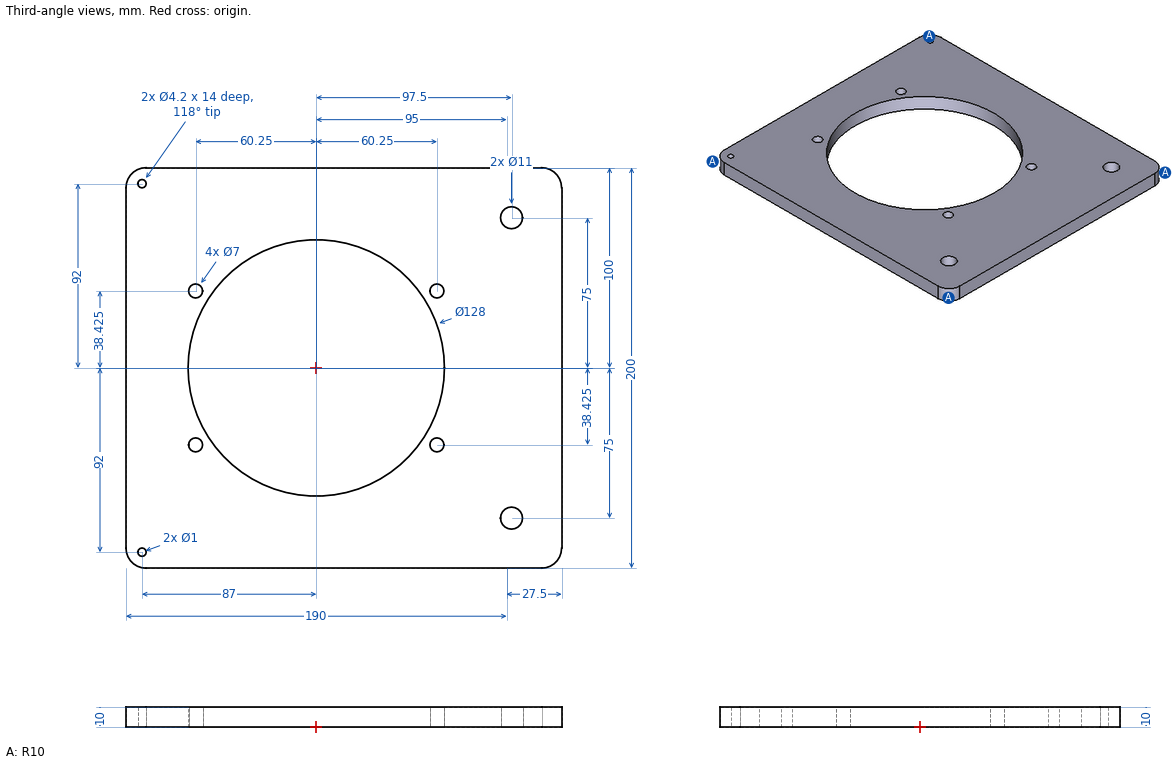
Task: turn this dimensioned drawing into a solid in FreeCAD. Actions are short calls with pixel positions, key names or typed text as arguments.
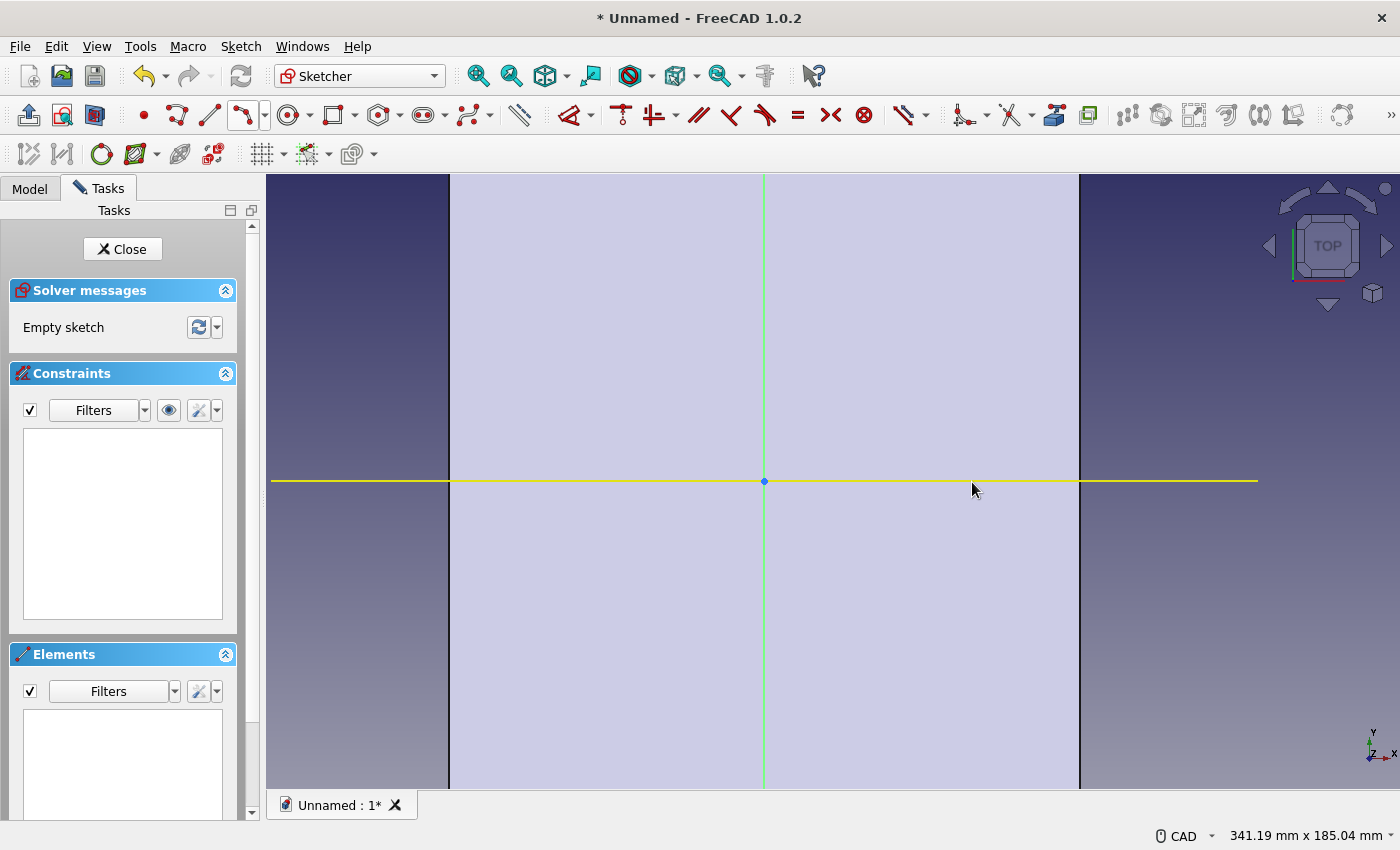
key(g)
key(c)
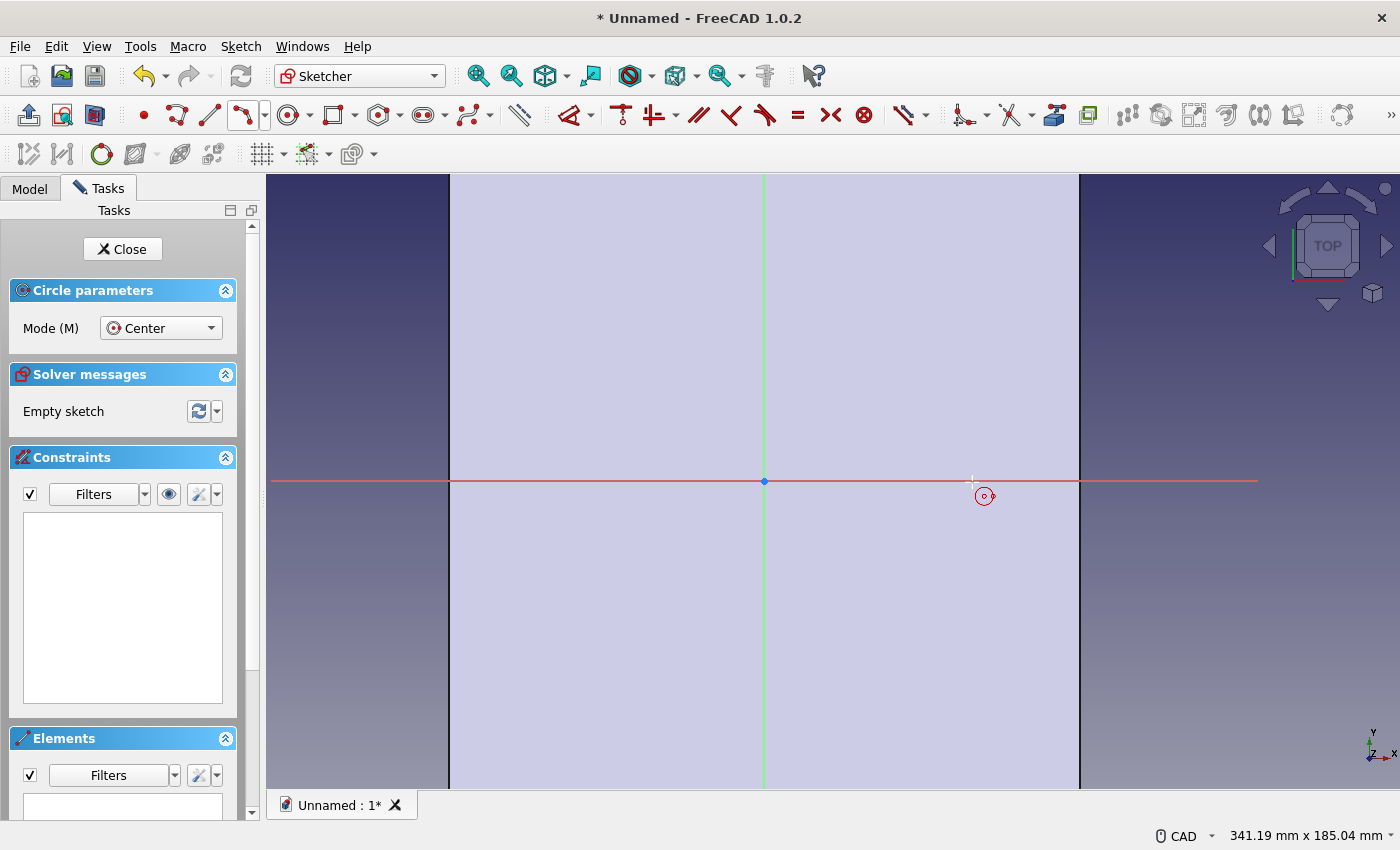
click(764, 481)
move(915, 331)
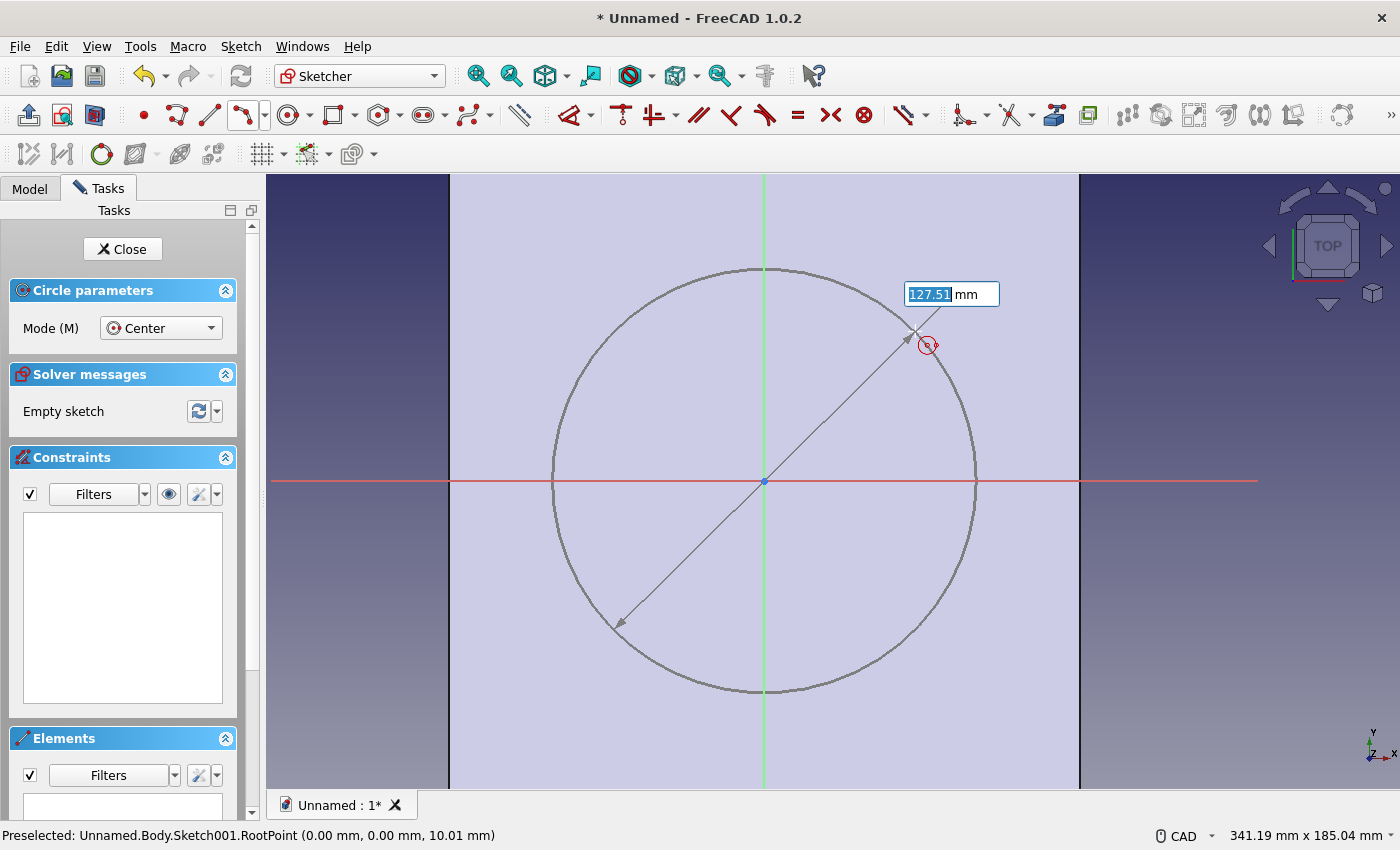
text(128)
key(Return)
key(Escape)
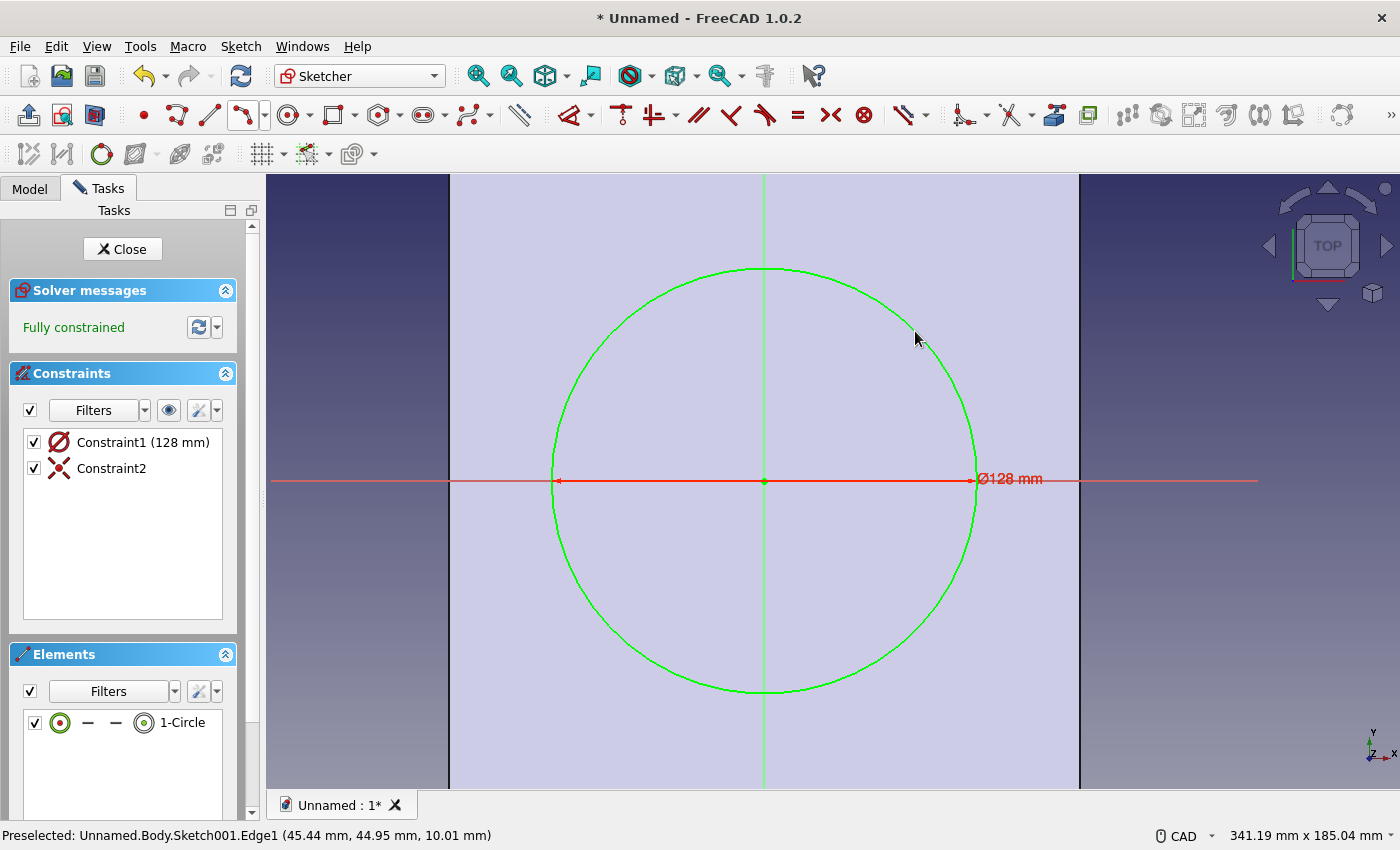
click(123, 249)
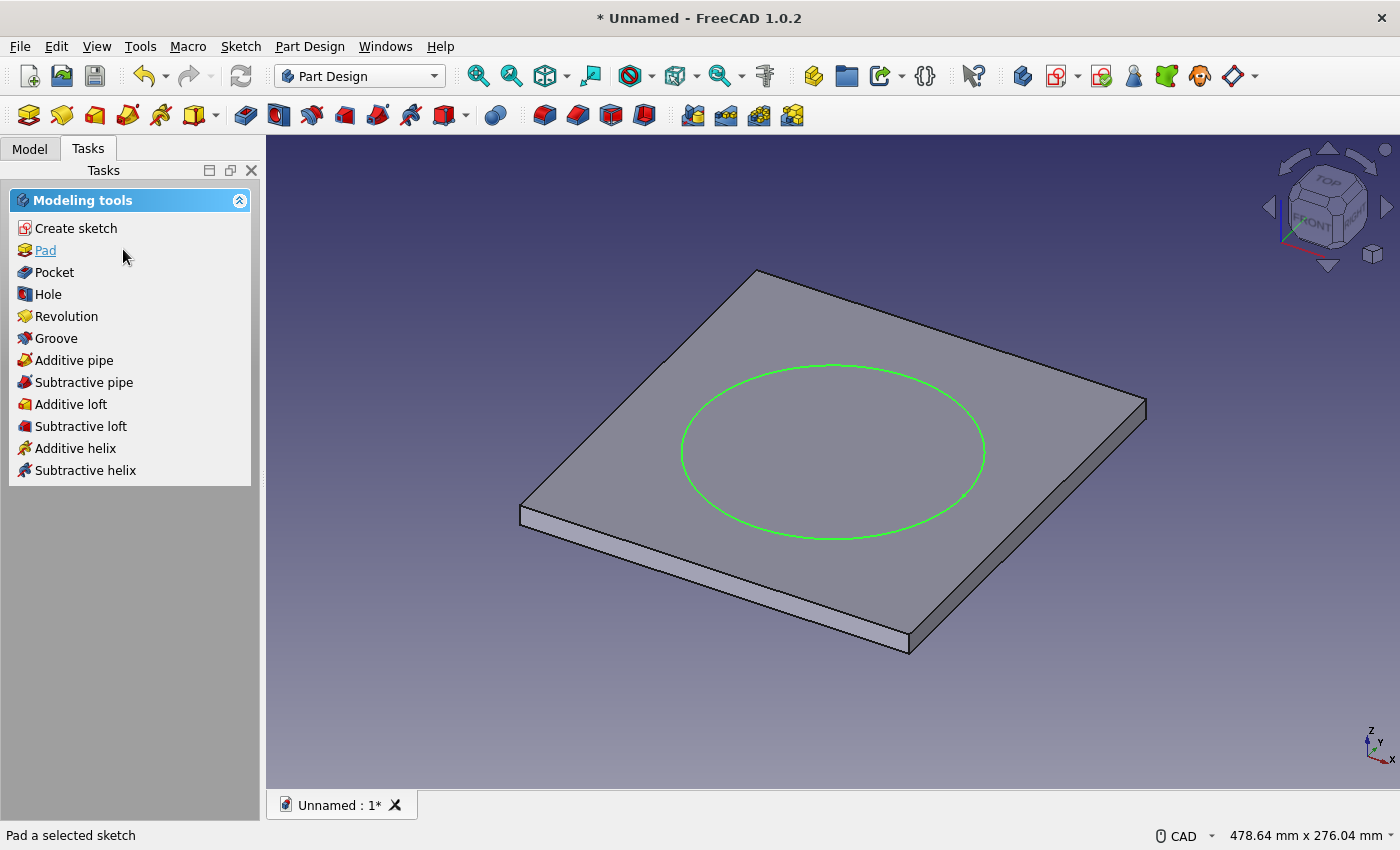
click(246, 116)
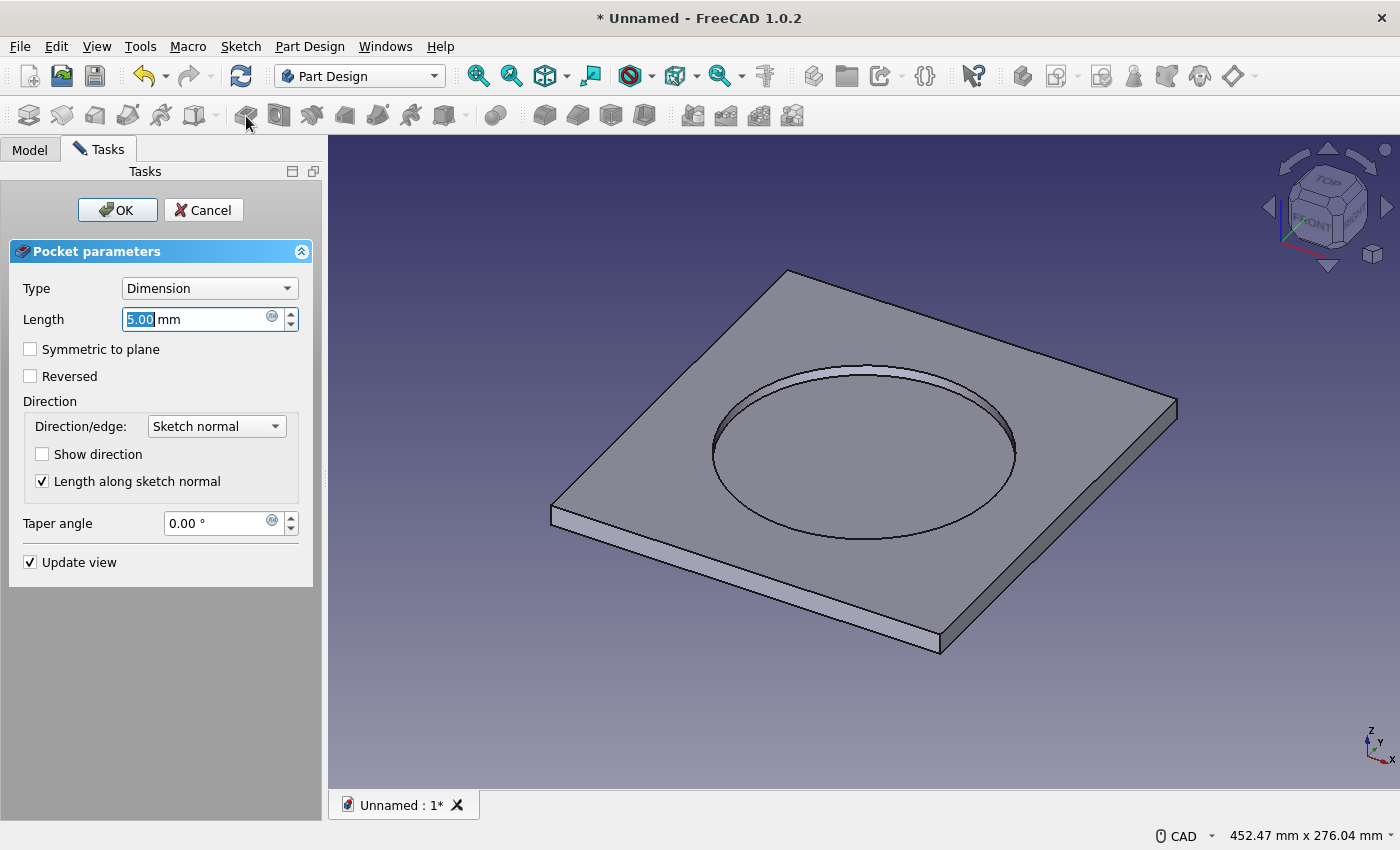
text(10)
key(Tab)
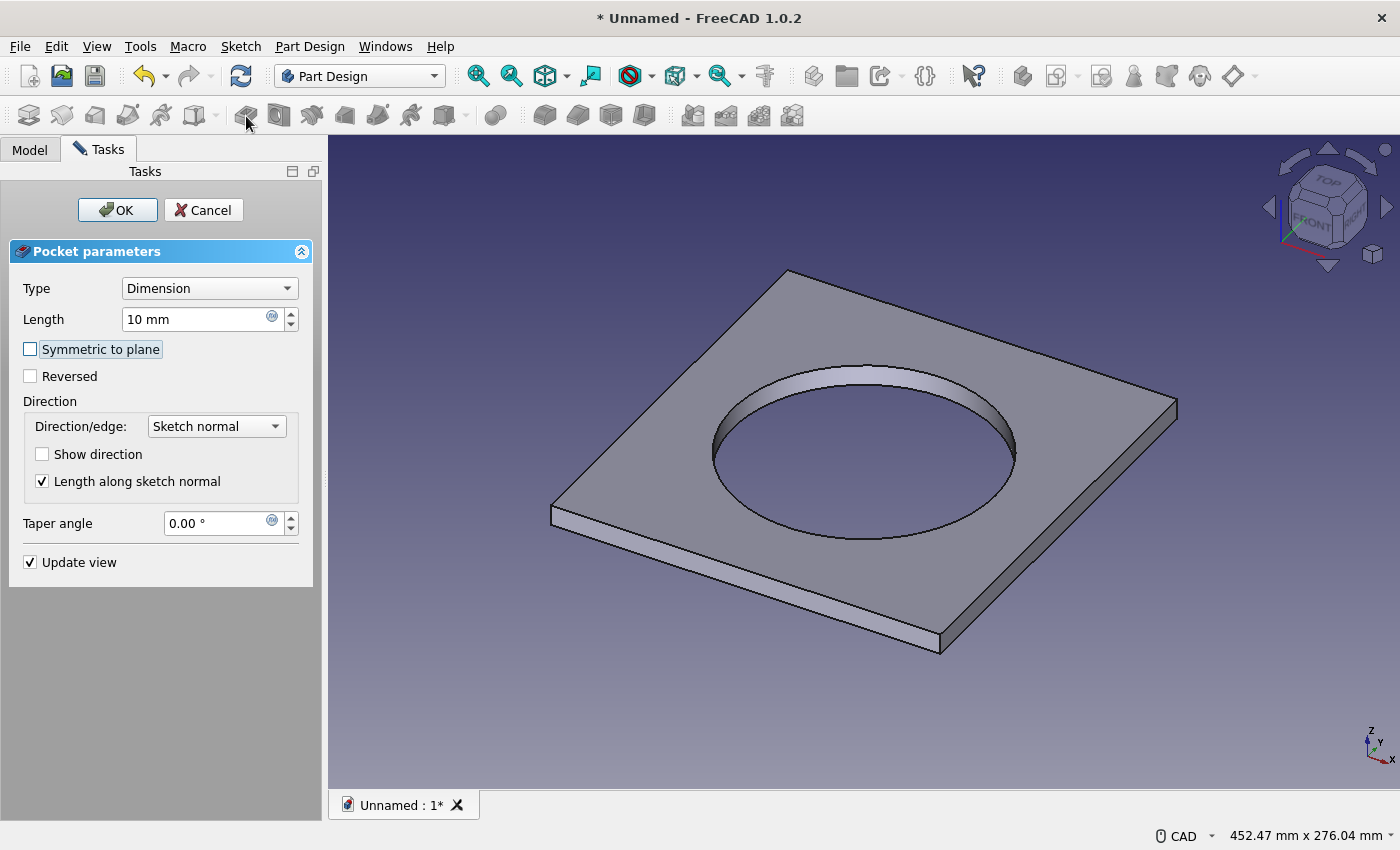
click(118, 210)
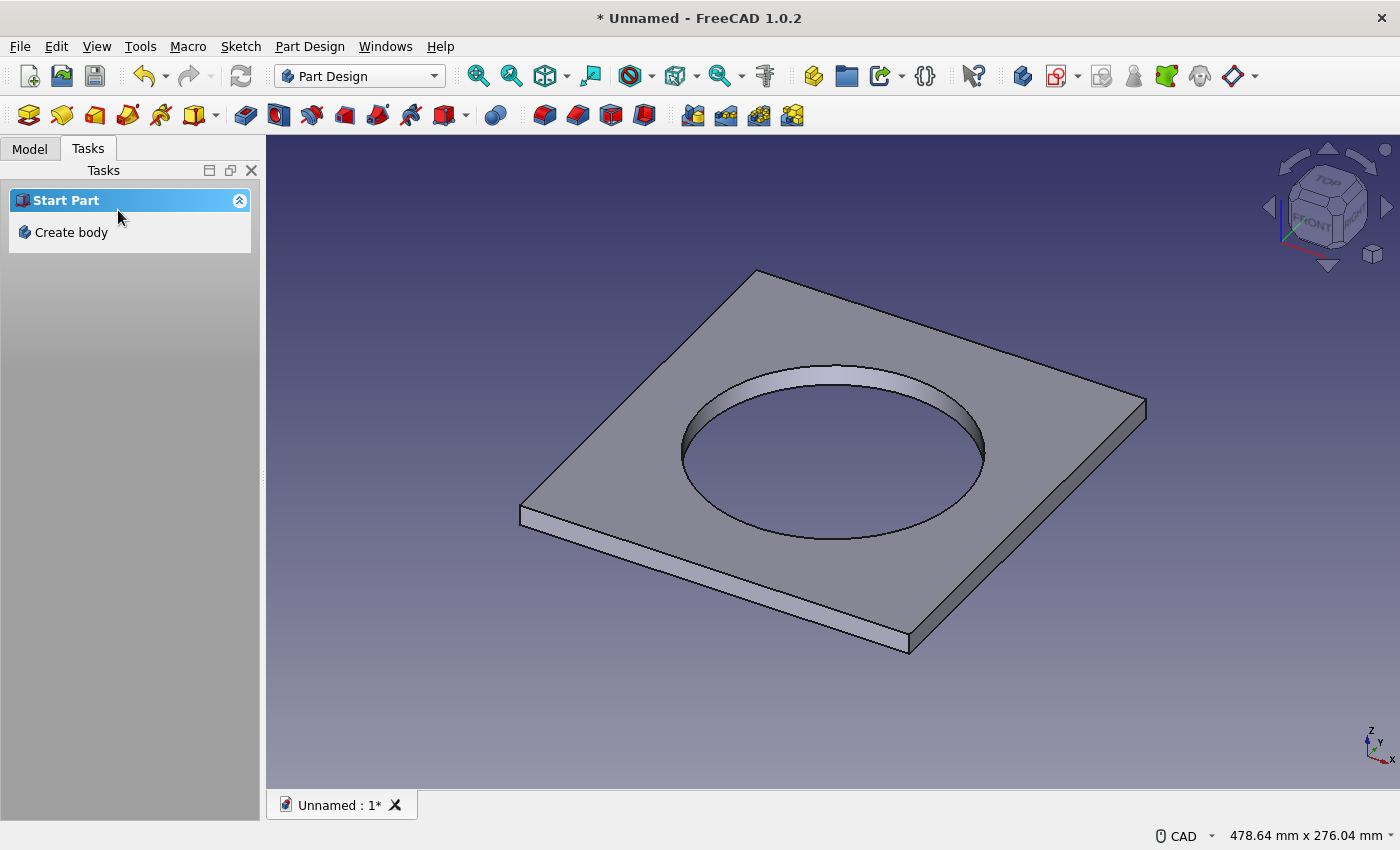
click(654, 482)